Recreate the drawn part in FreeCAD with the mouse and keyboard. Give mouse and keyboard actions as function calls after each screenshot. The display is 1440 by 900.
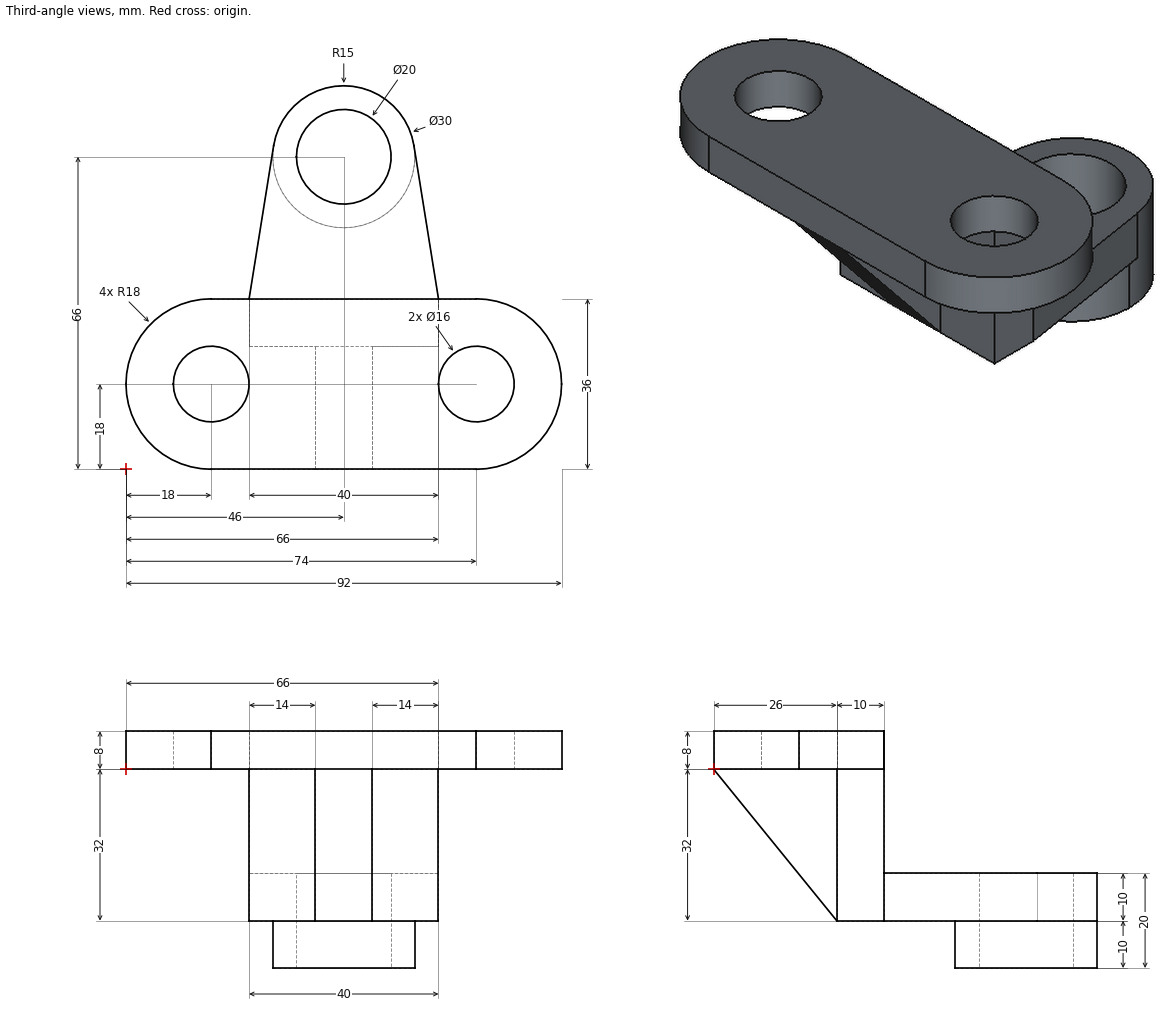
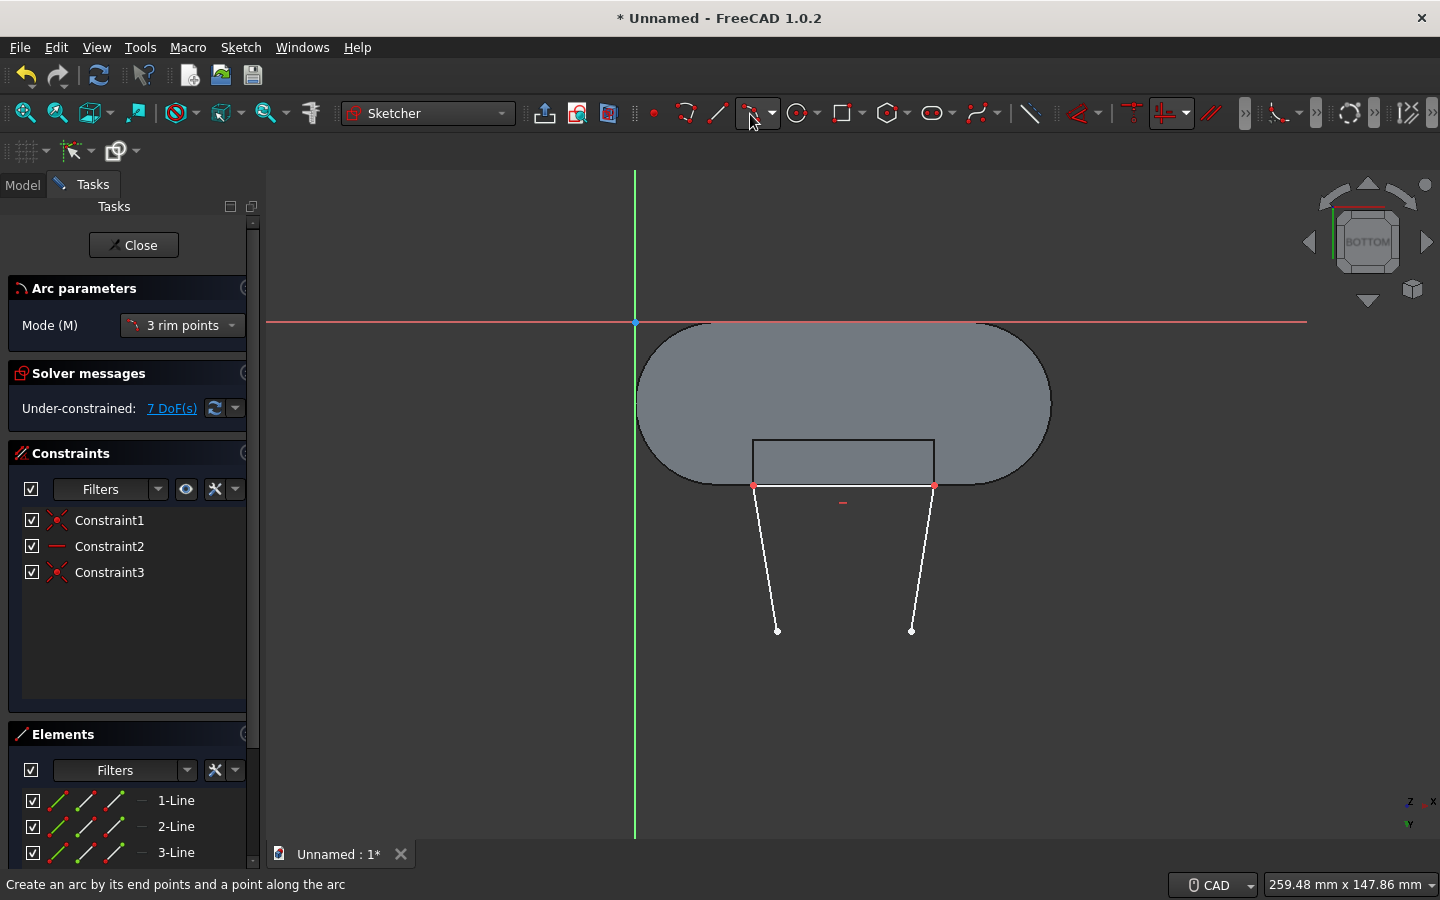
click(777, 632)
click(911, 632)
click(844, 689)
key(Escape)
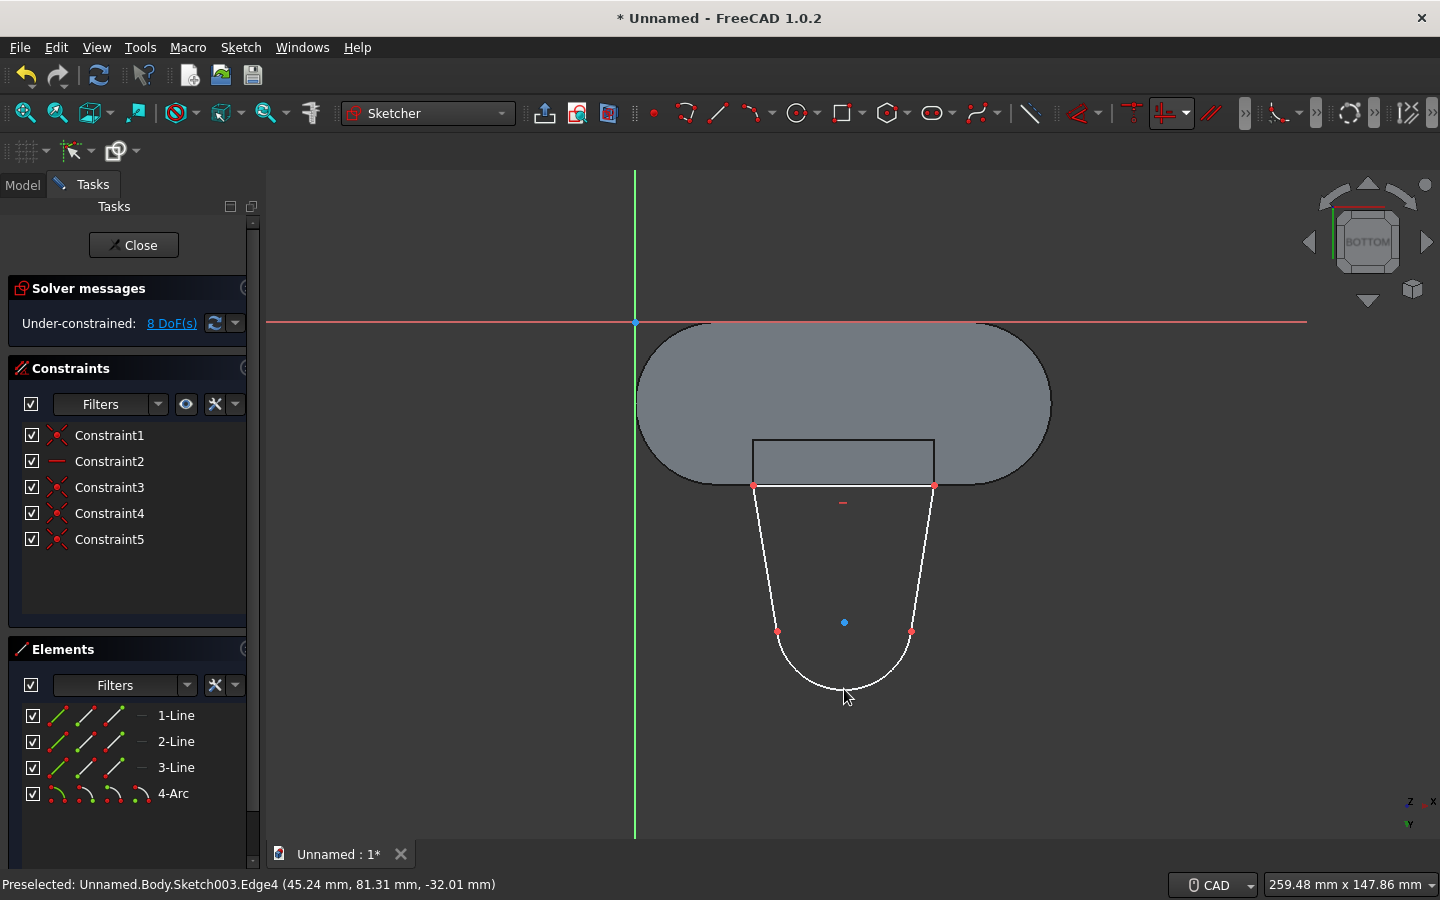
click(918, 588)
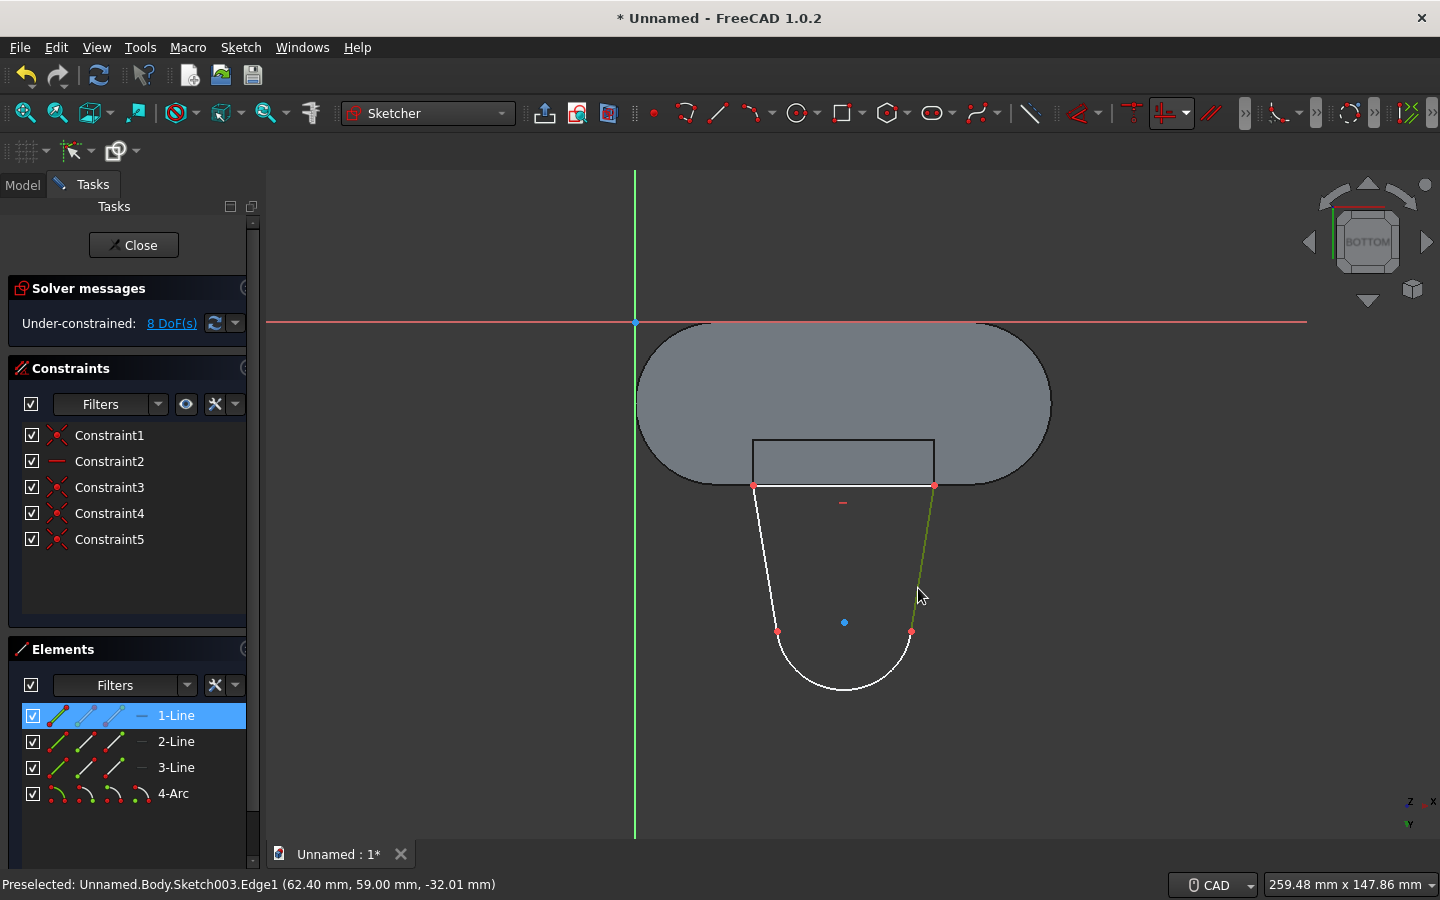
click(807, 679)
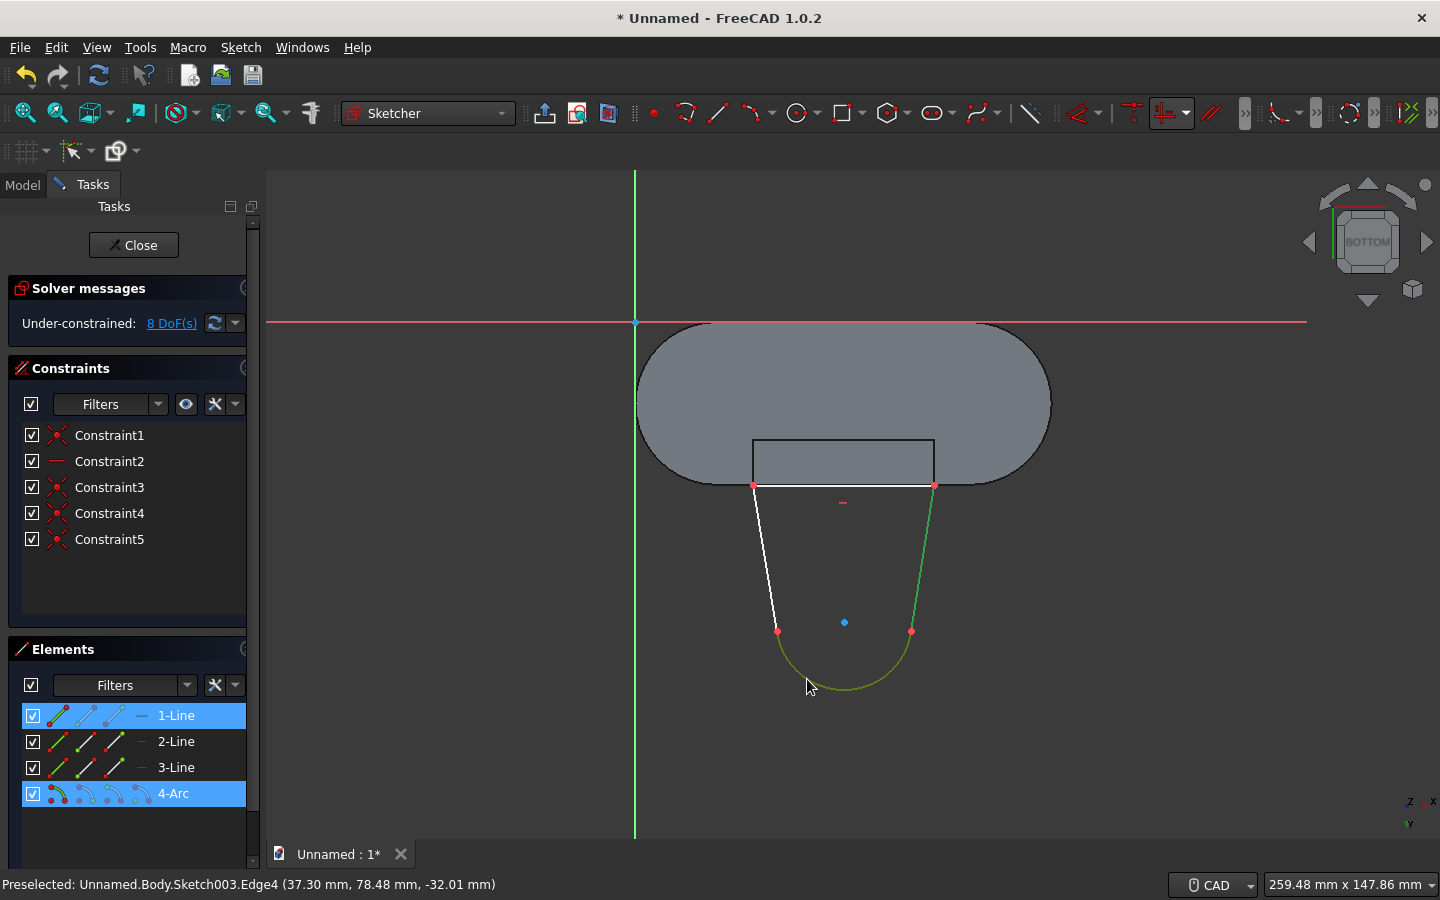
key(t)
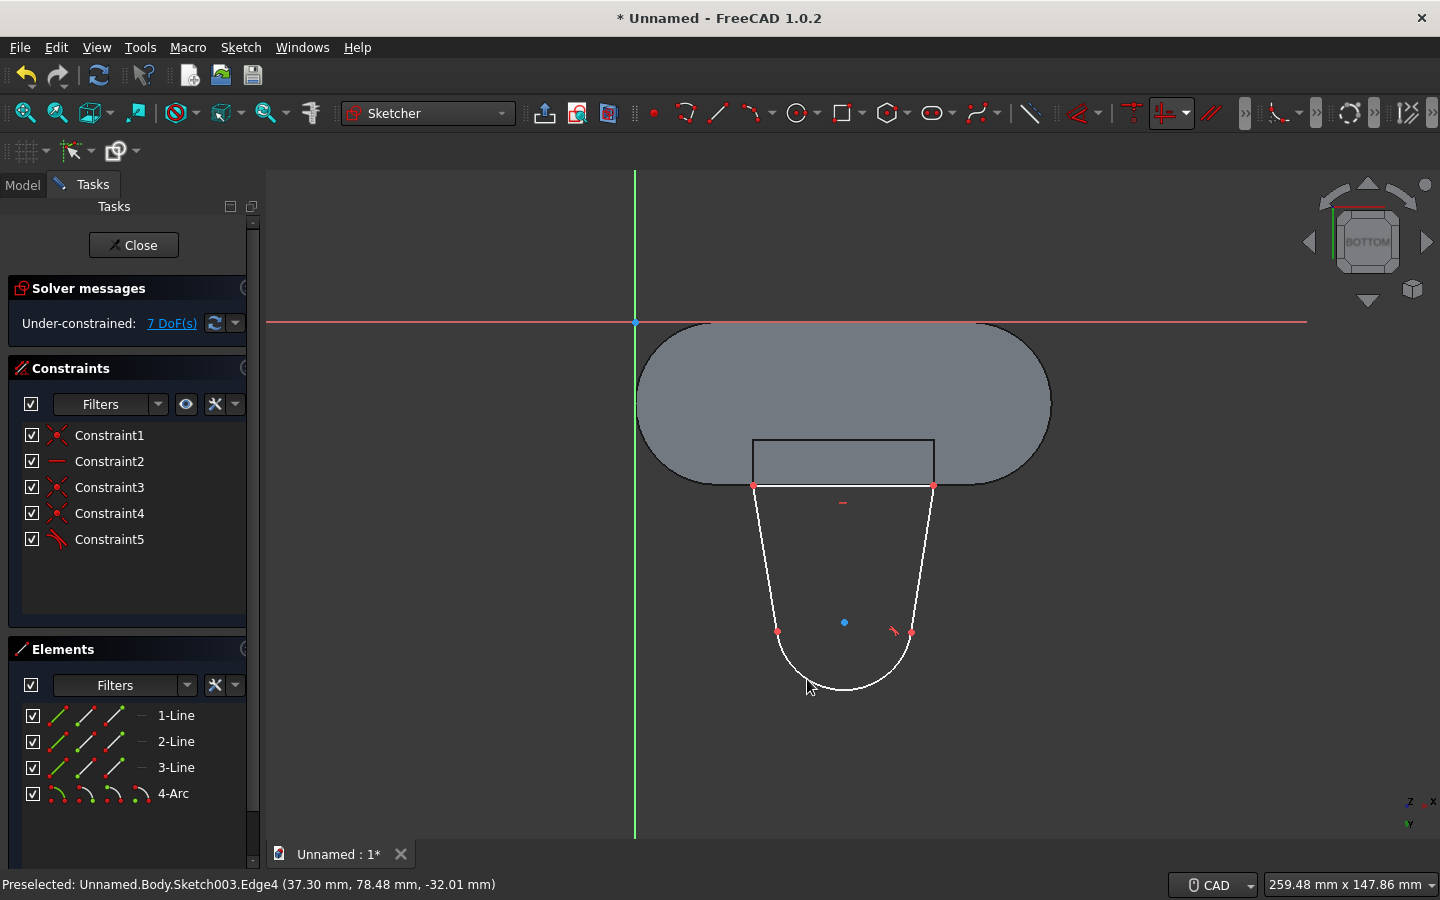
click(760, 530)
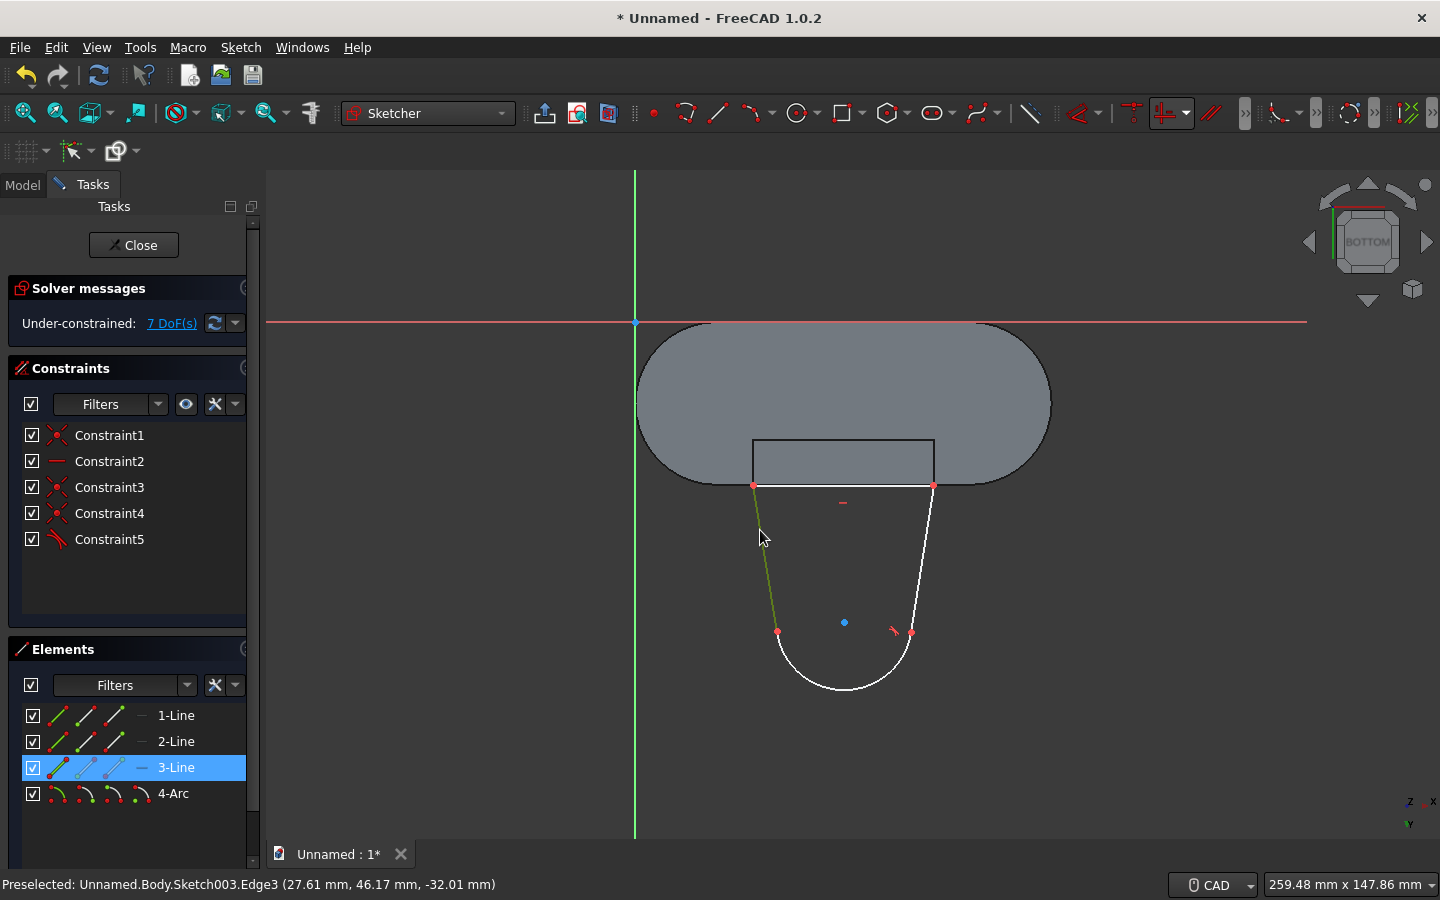
click(807, 679)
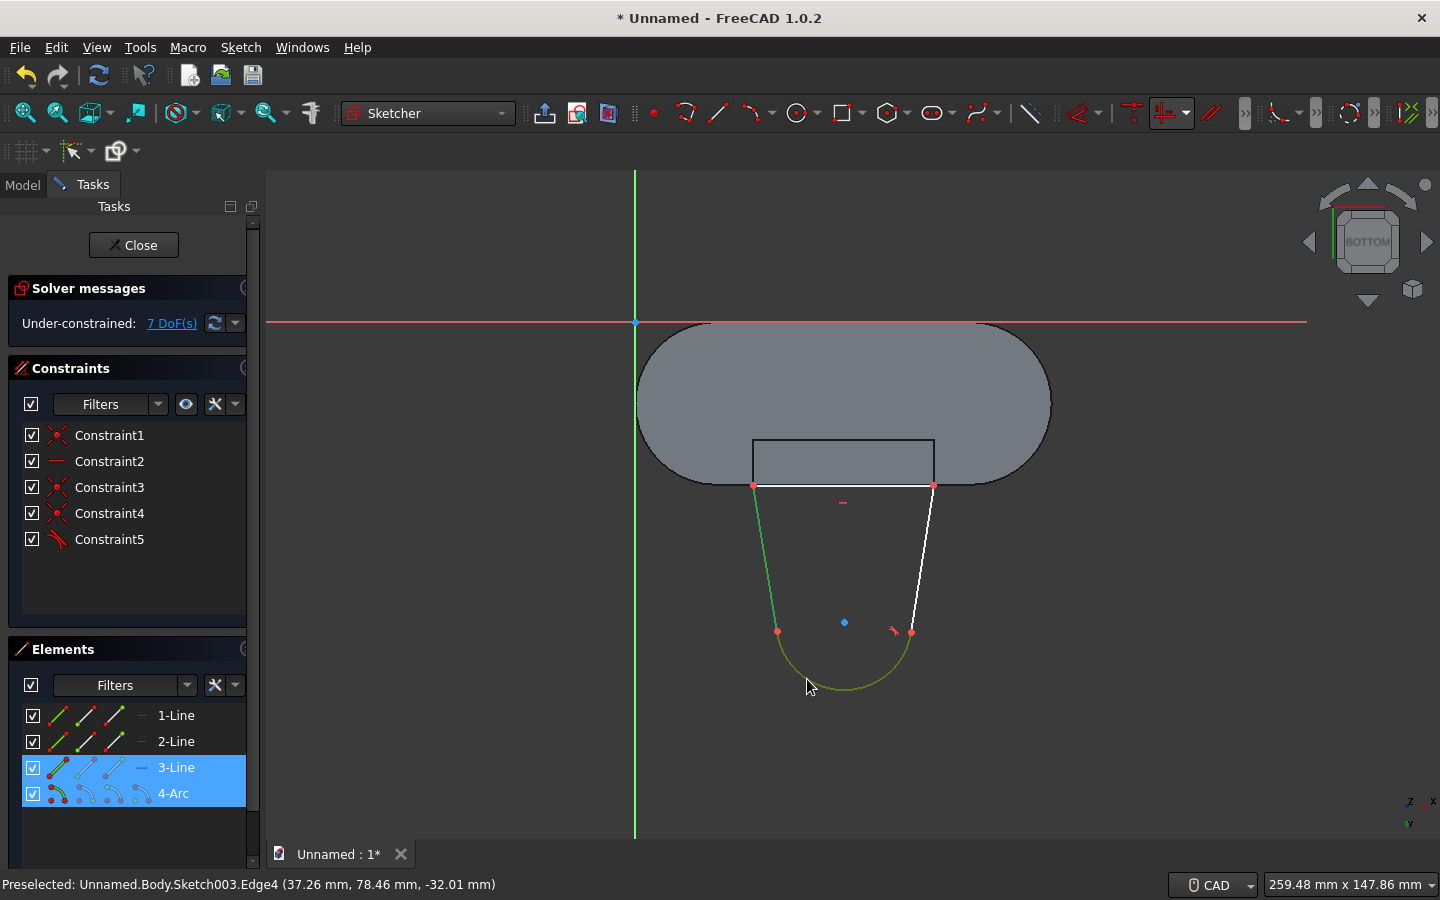
key(t)